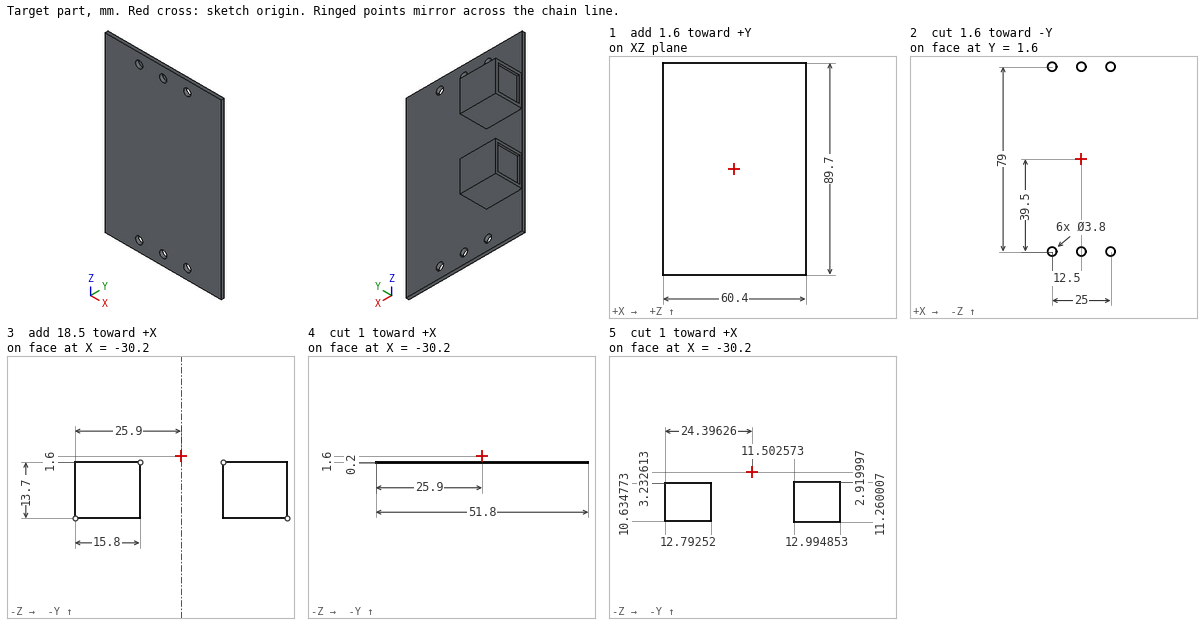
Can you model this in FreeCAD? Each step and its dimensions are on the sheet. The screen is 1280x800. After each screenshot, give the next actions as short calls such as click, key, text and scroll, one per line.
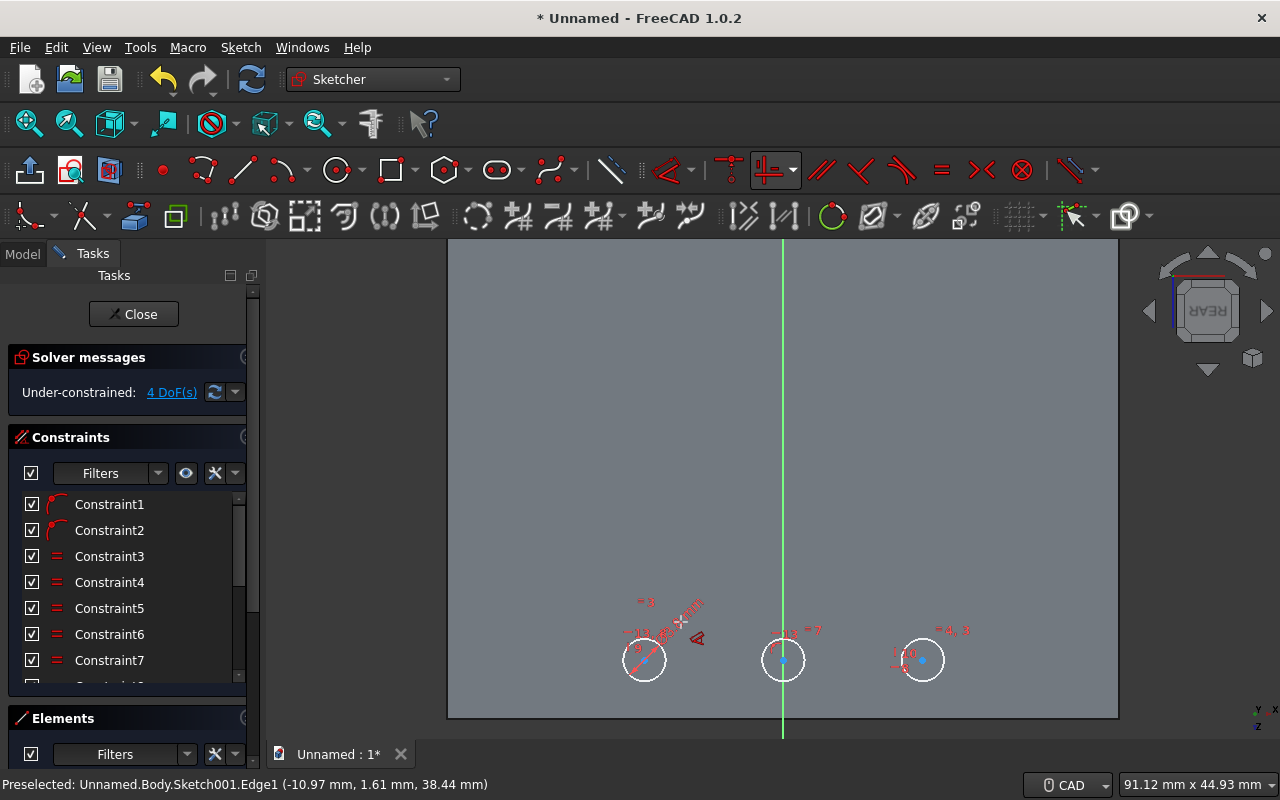
click(644, 660)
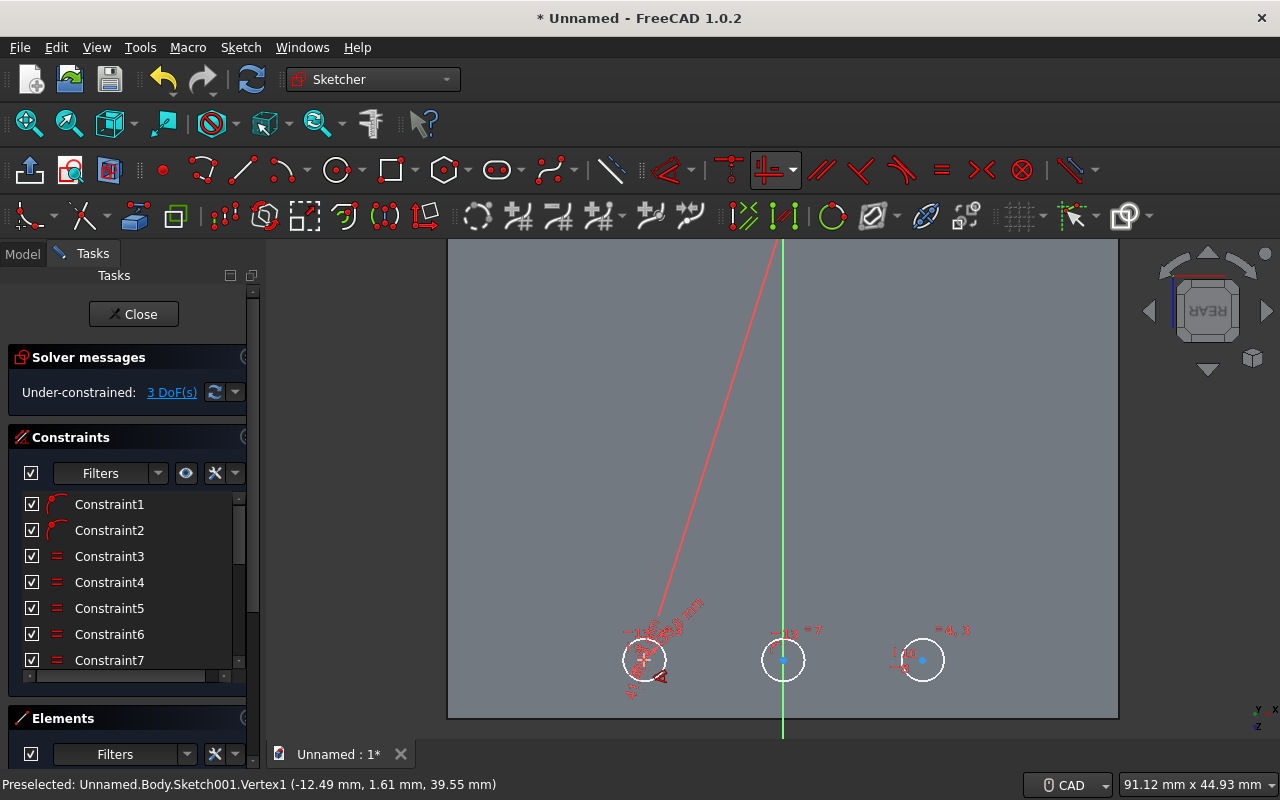
click(923, 660)
click(720, 694)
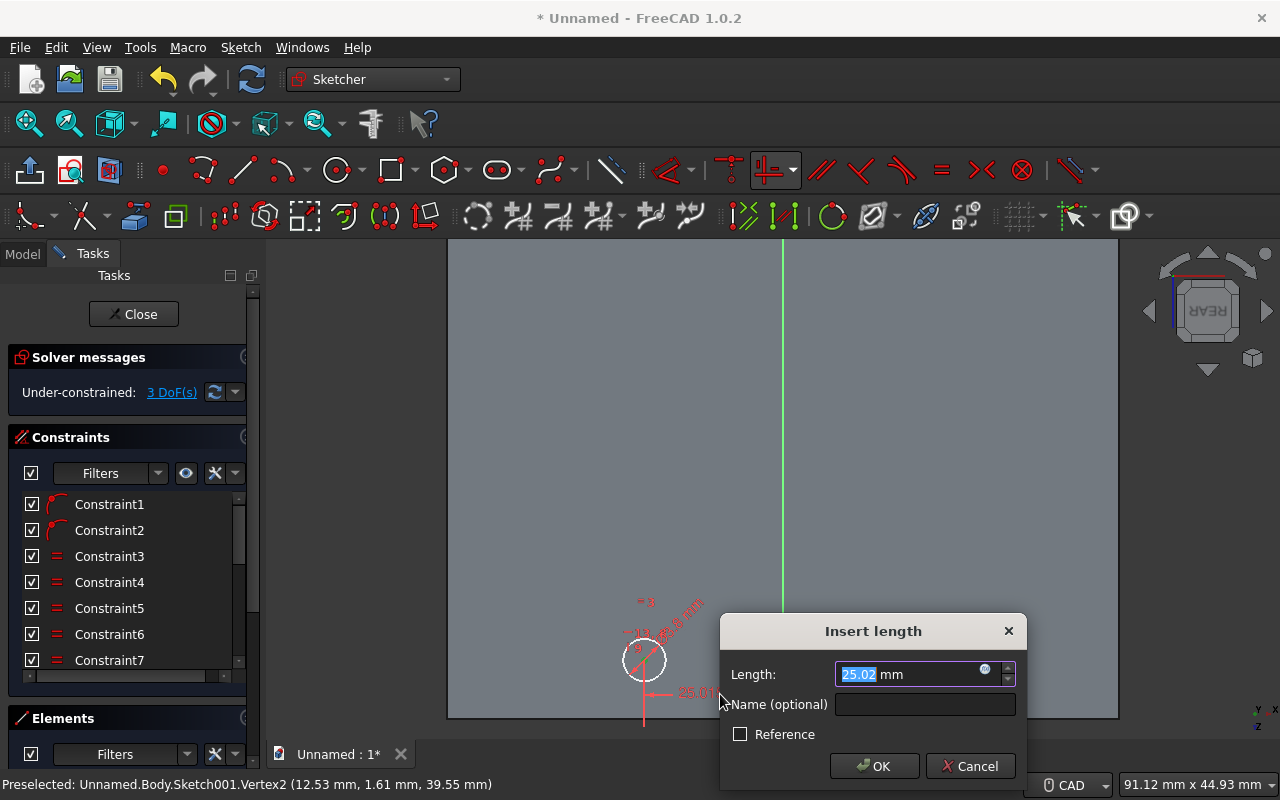
text(25)
key(Return)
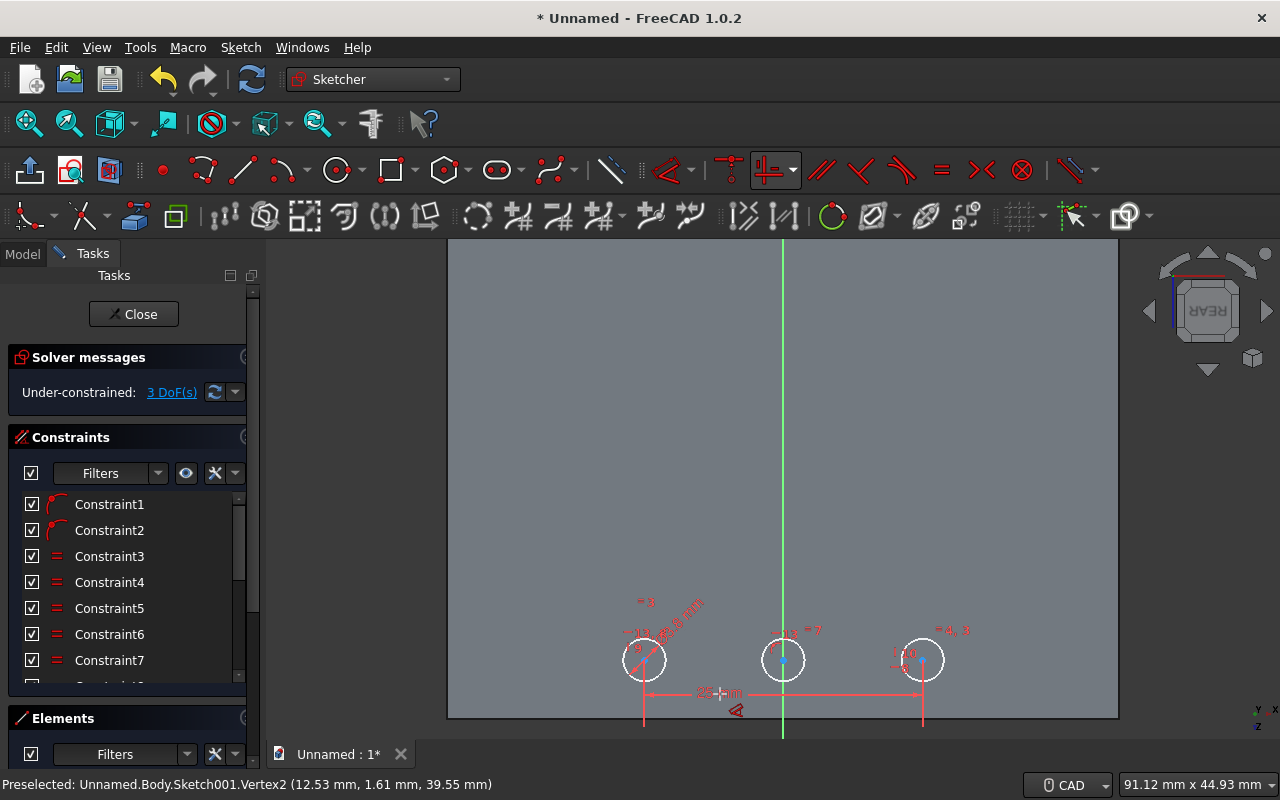
click(644, 660)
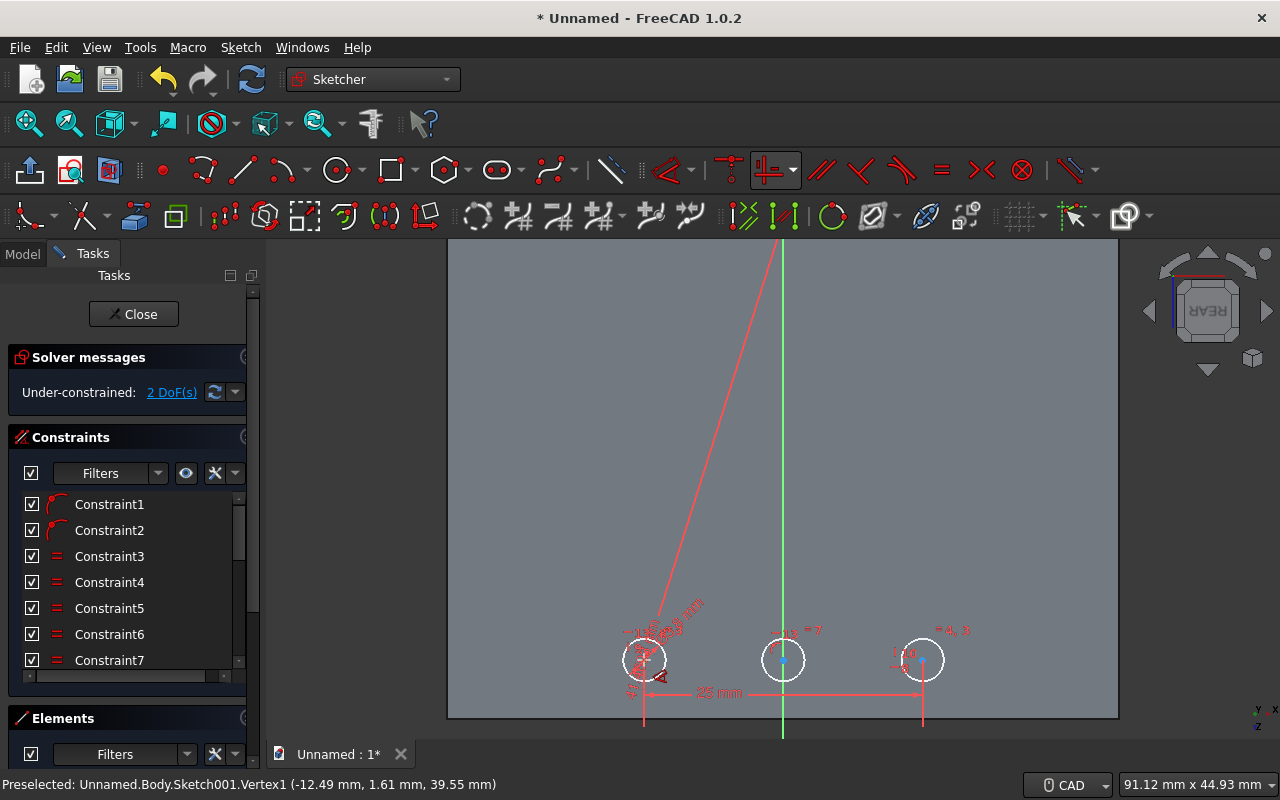
scroll(659, 646, down, 5)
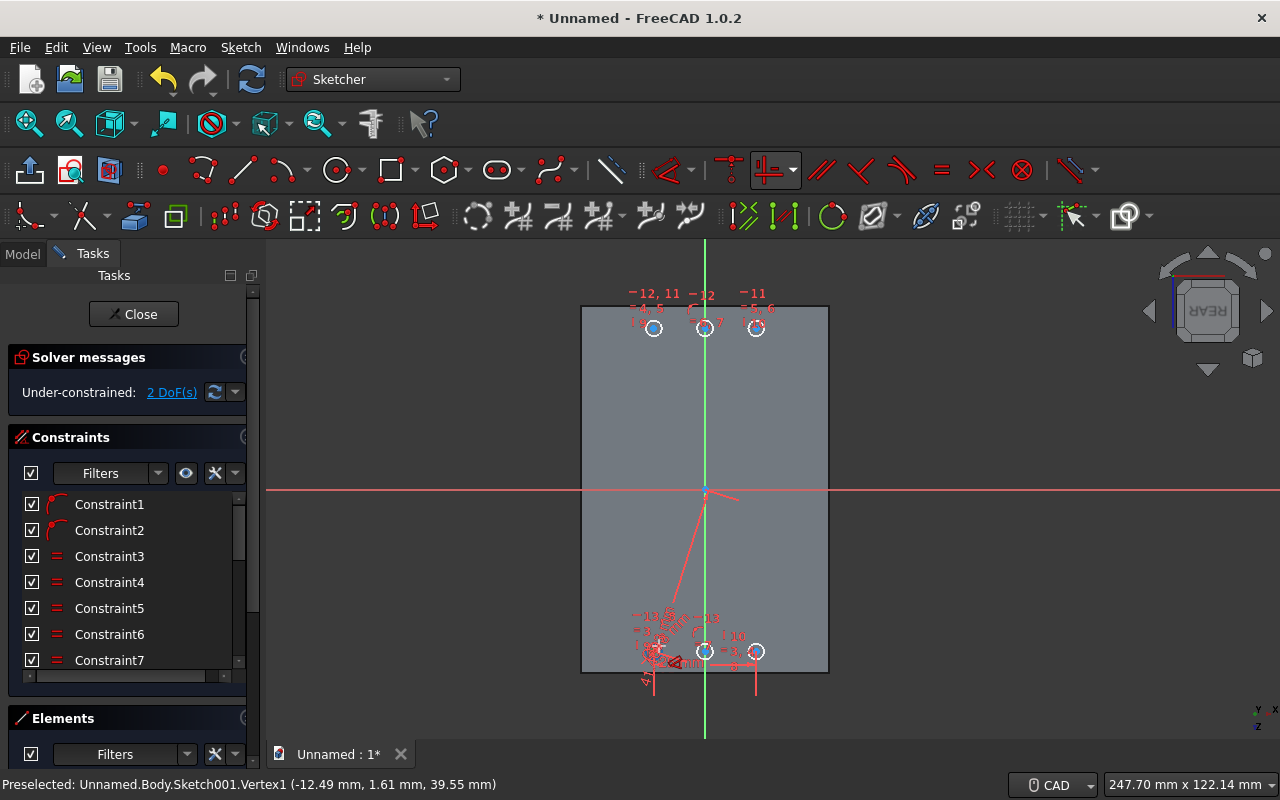
click(654, 328)
click(620, 416)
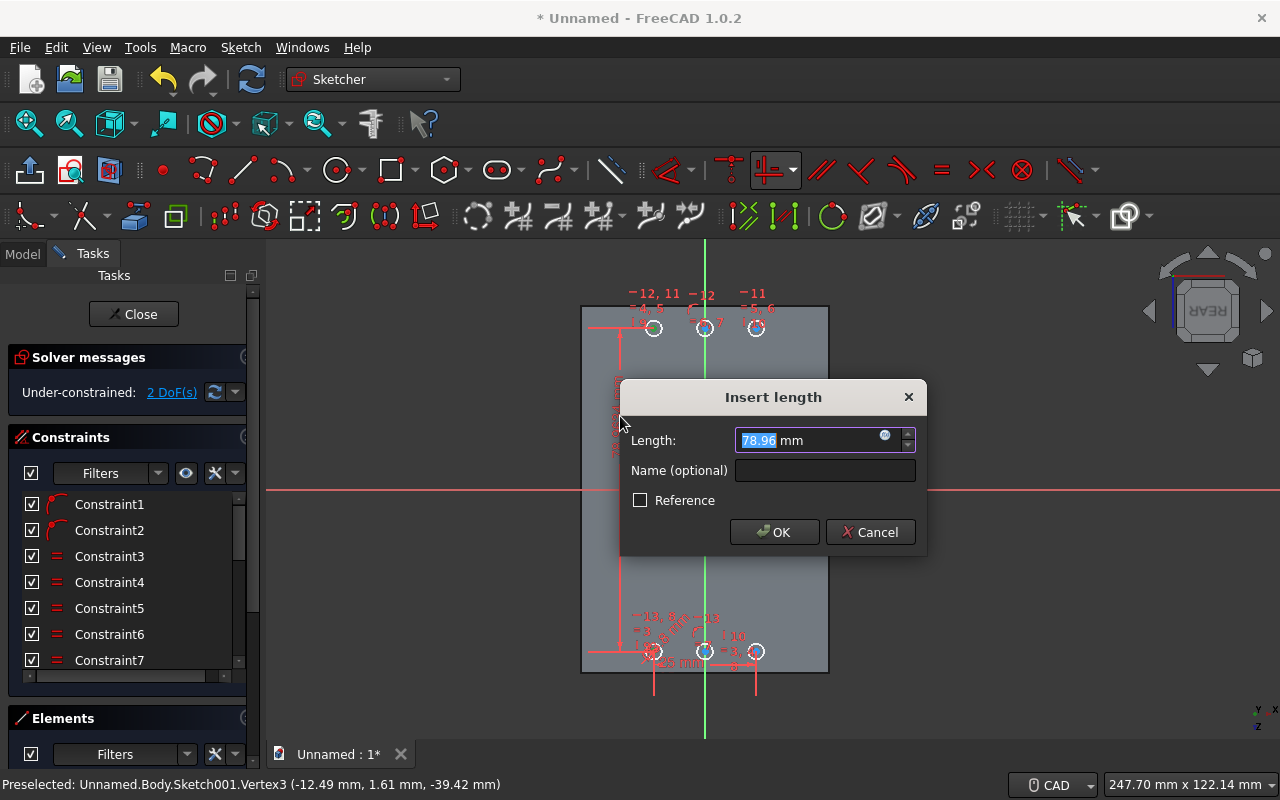
text(79)
key(Return)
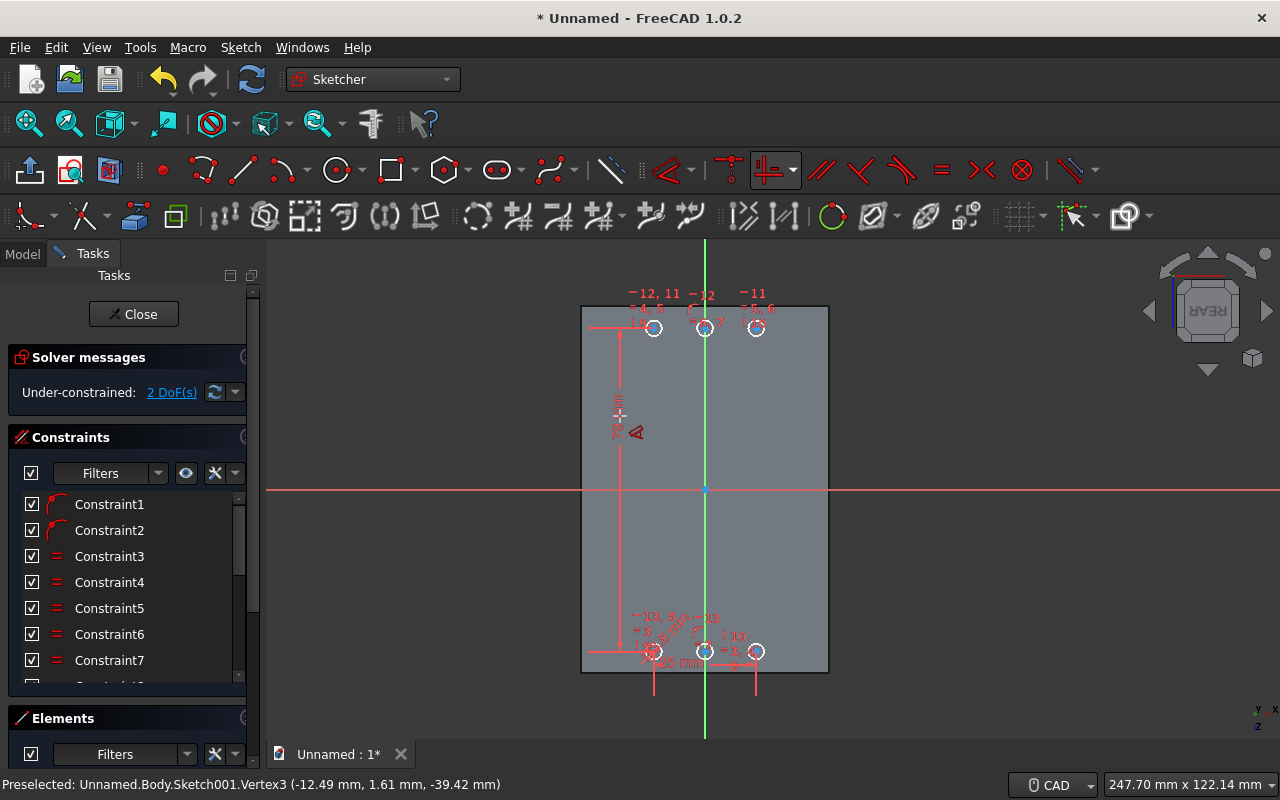
click(654, 652)
click(679, 686)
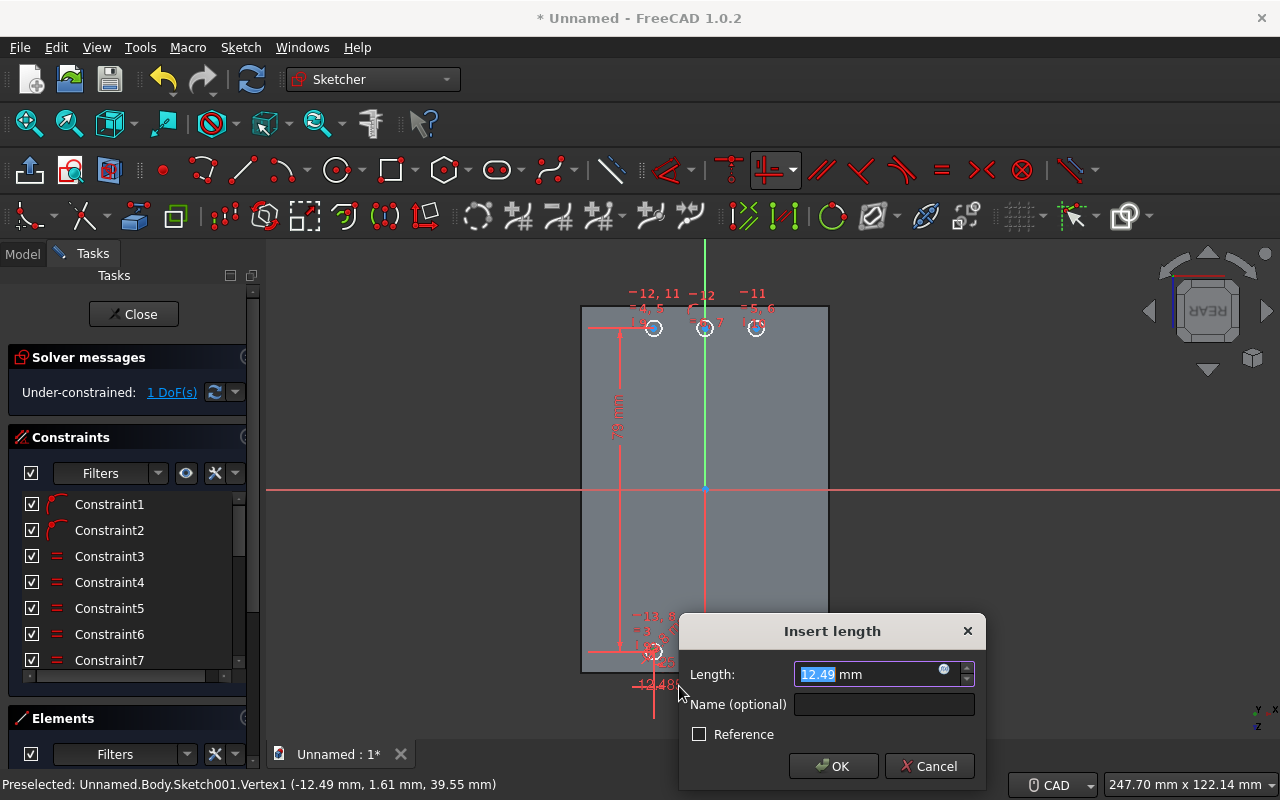
text(12.5)
key(Return)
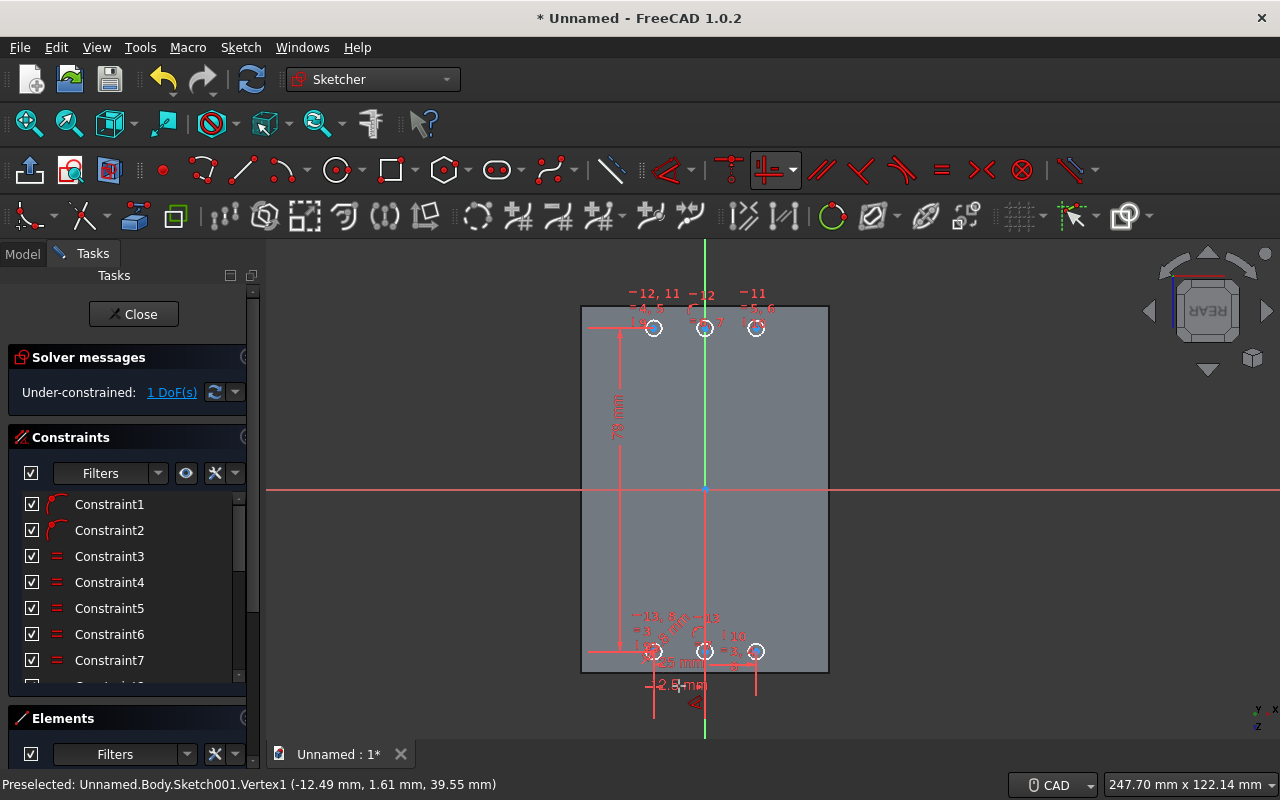
click(654, 652)
click(620, 571)